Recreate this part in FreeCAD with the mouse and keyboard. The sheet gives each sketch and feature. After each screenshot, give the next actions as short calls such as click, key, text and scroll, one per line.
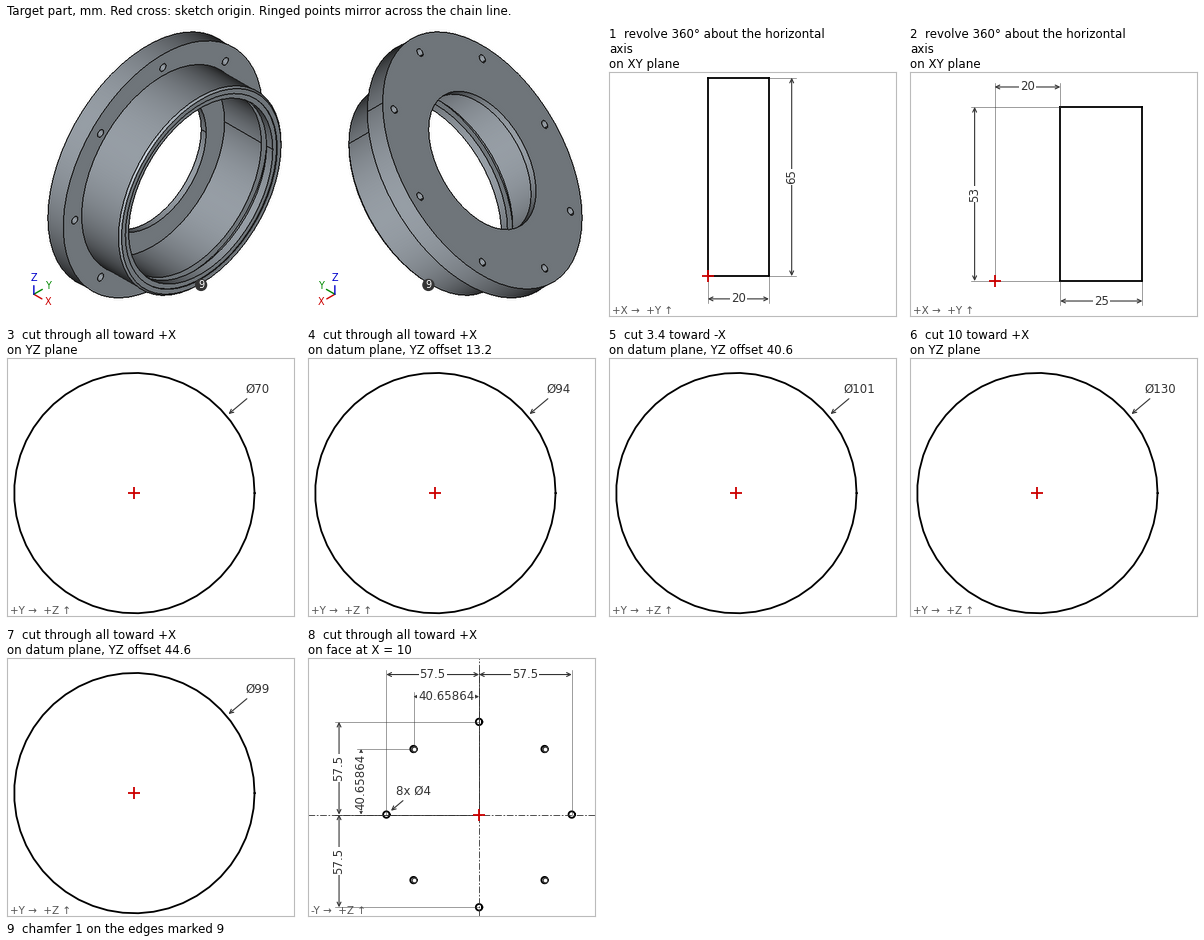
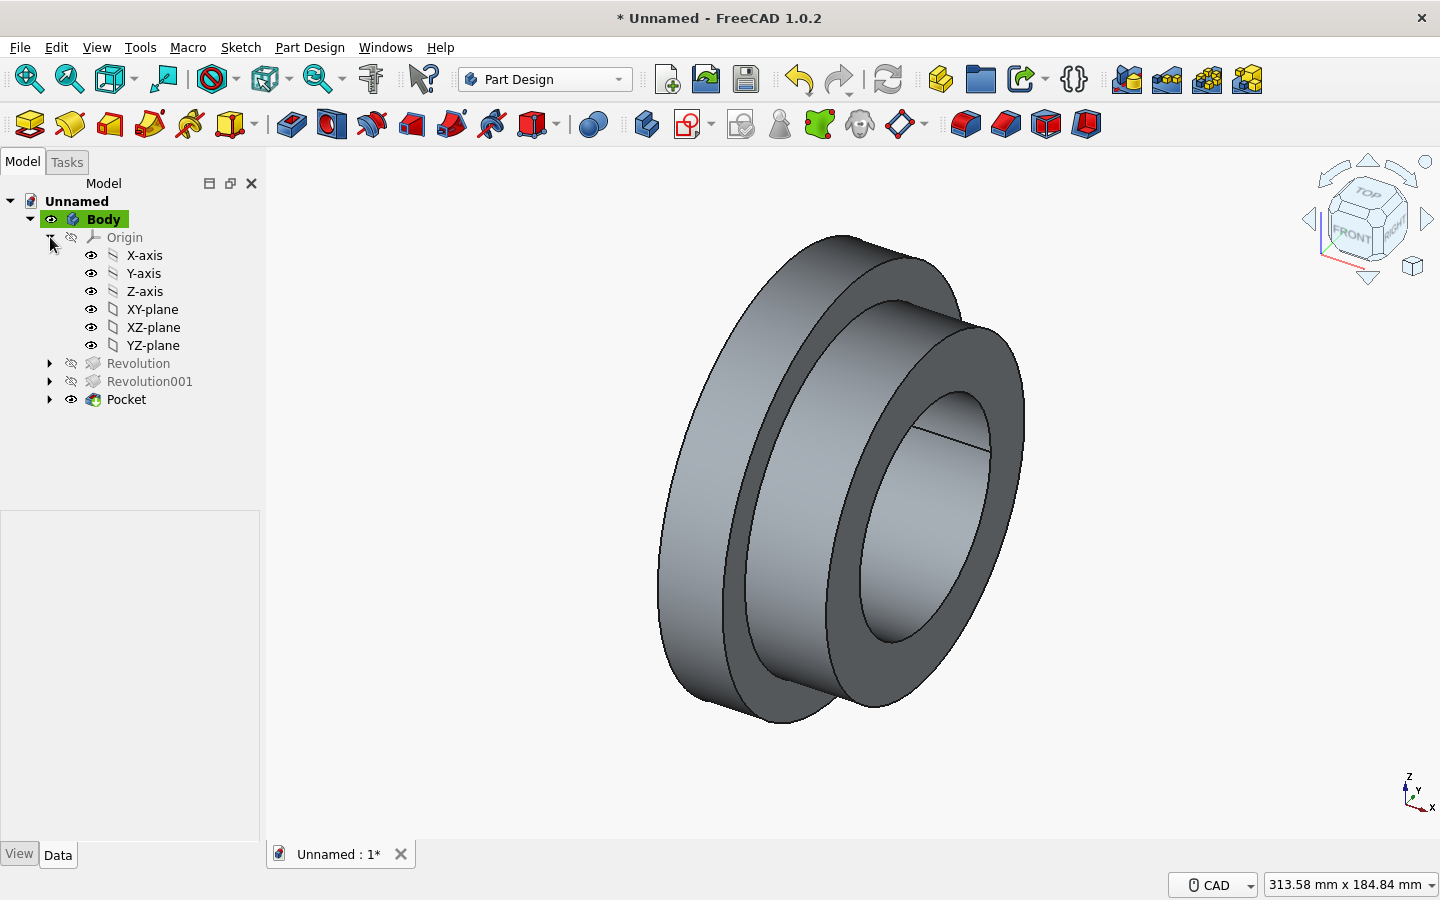
click(136, 345)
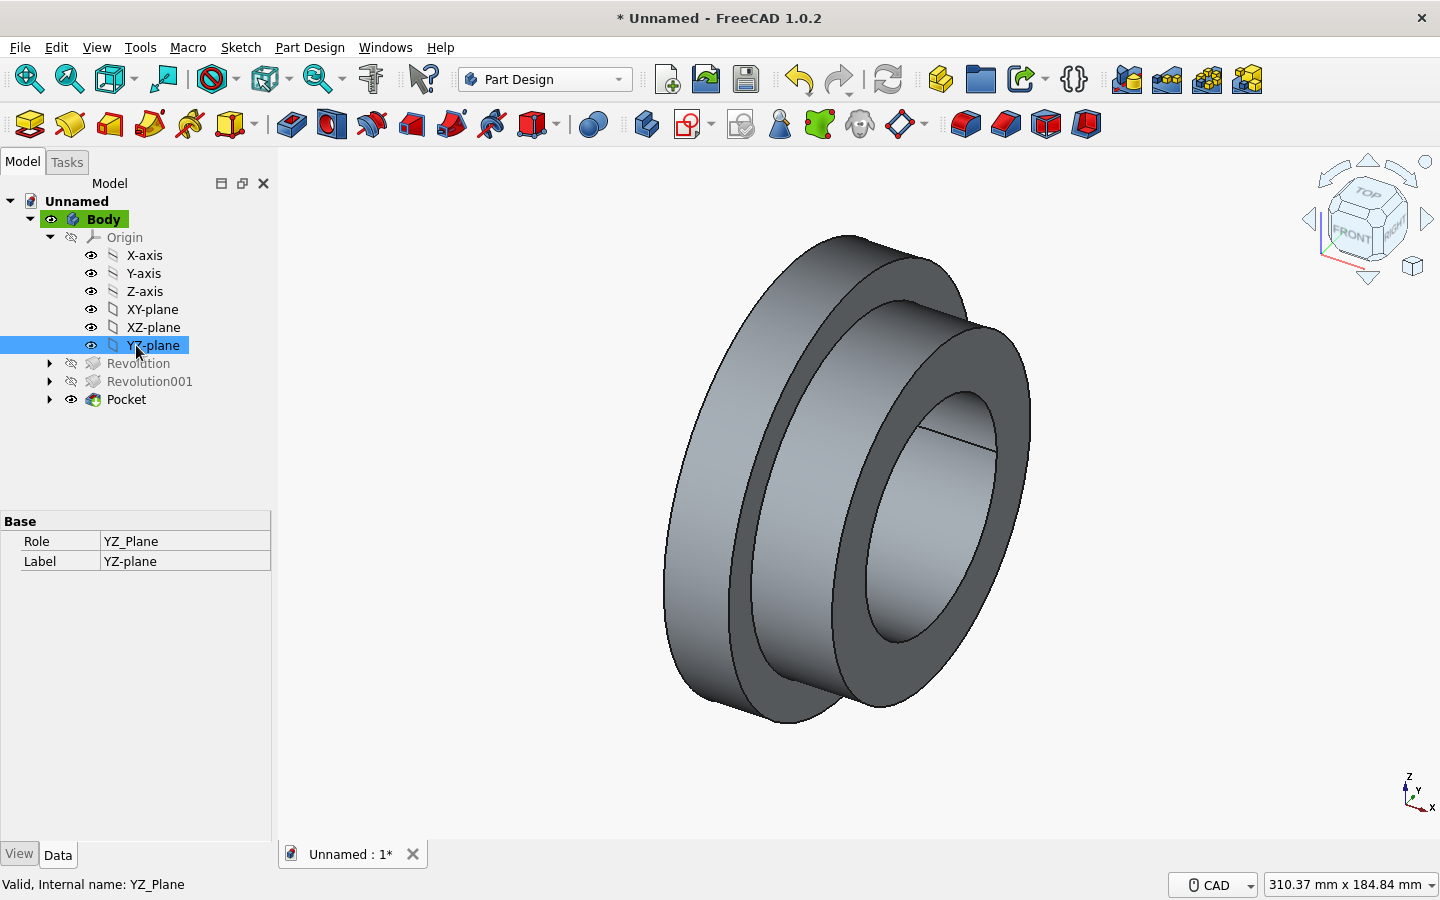
click(900, 124)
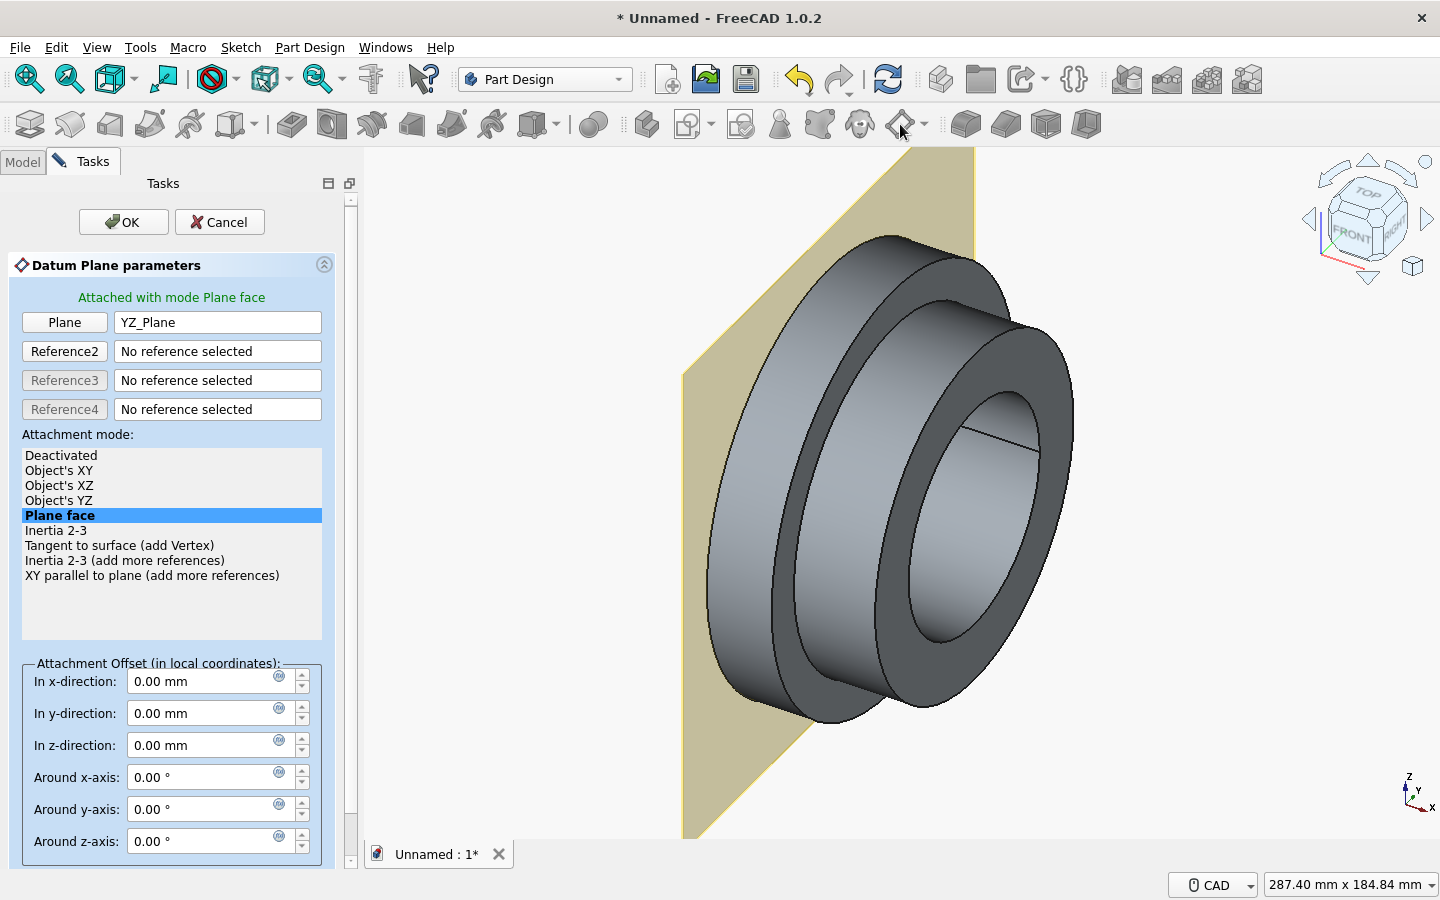
triple_click(210, 745)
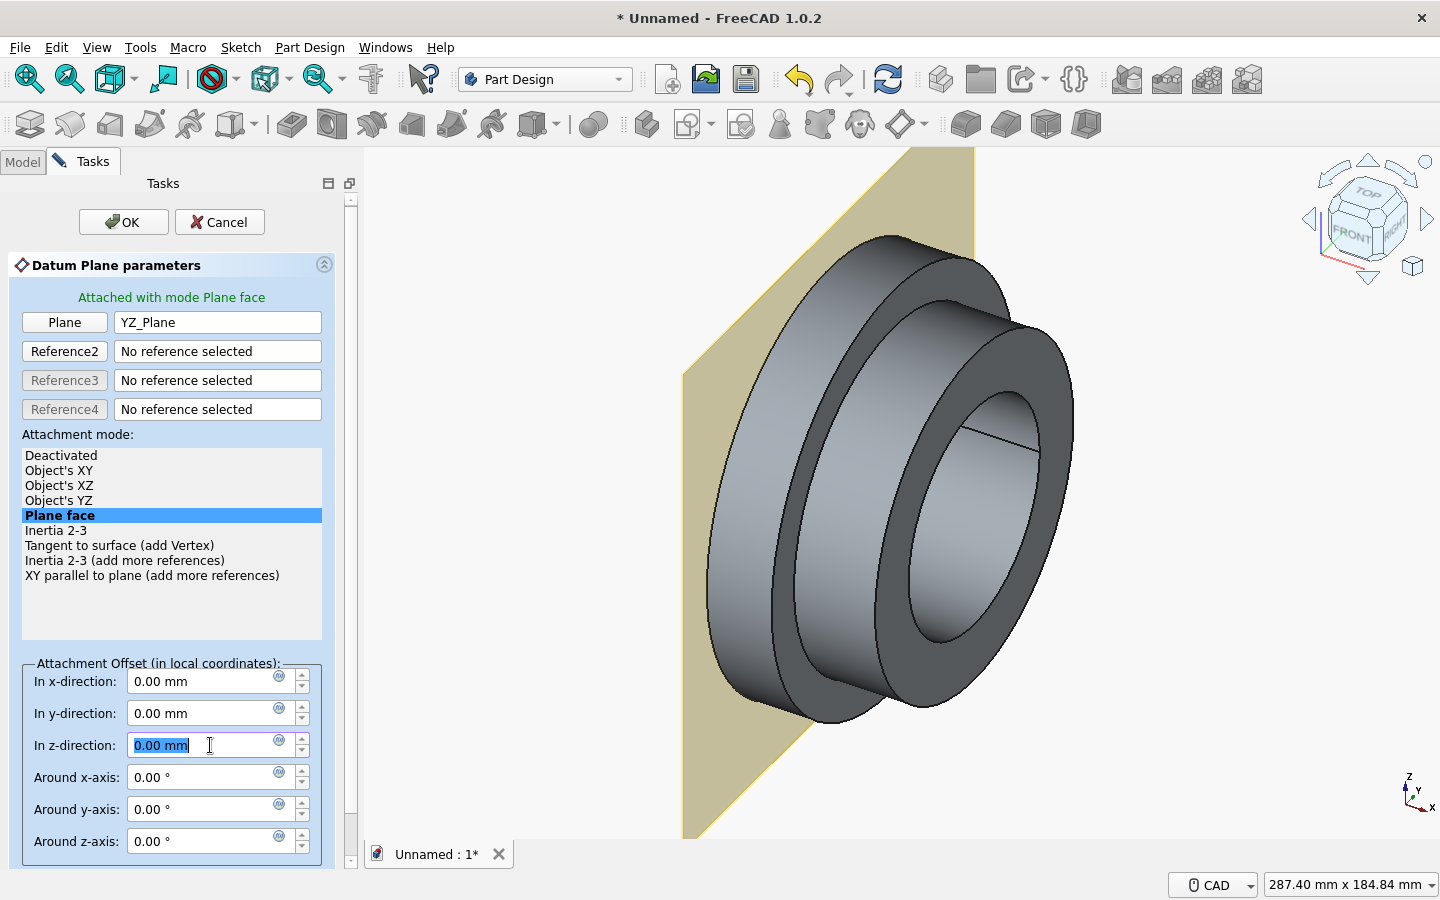
text(13.2)
key(Tab)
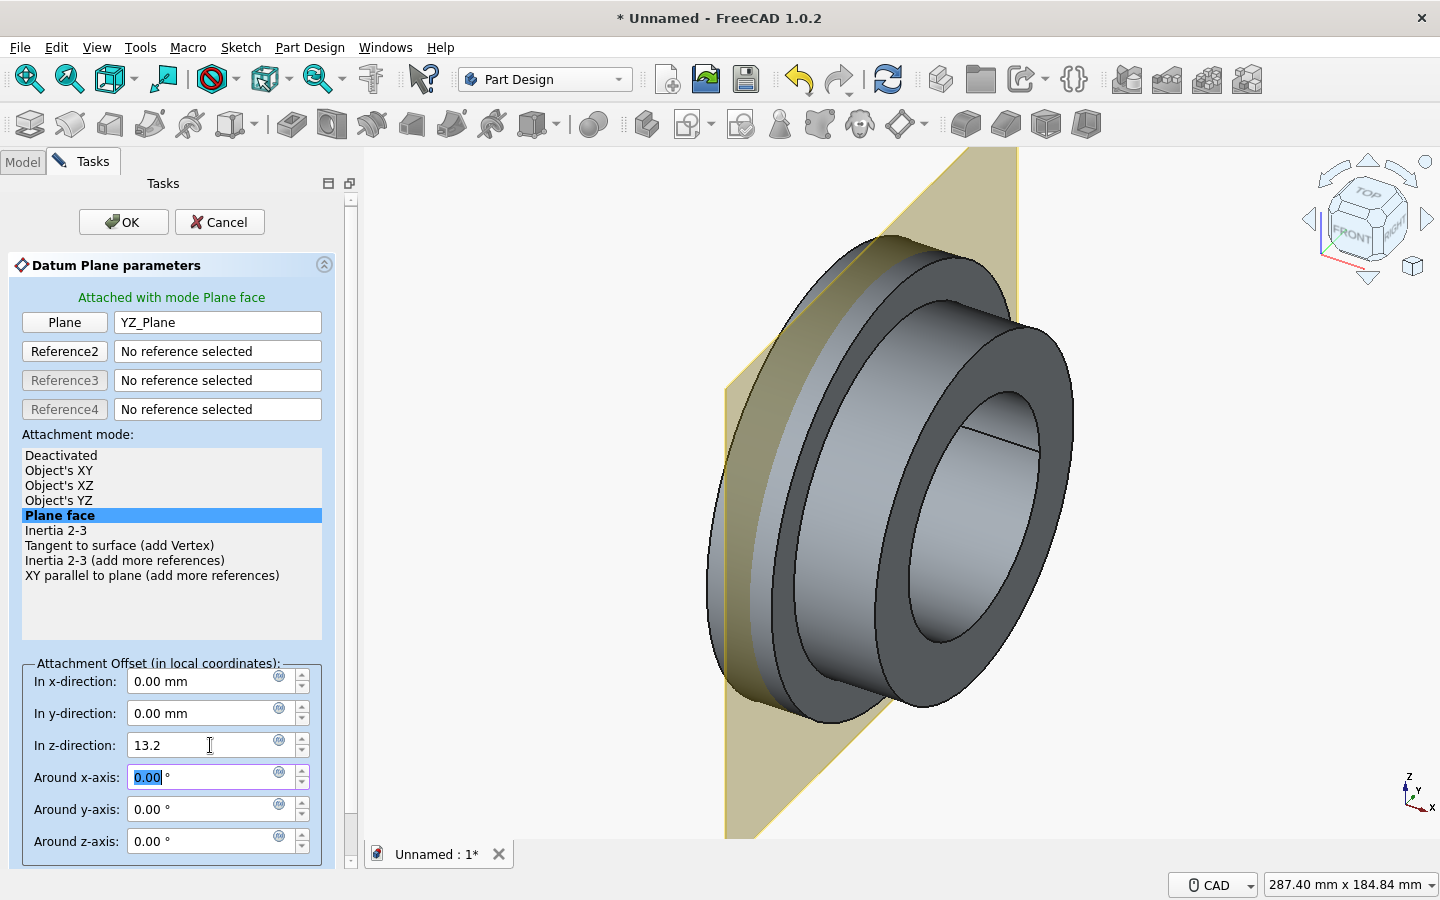
click(124, 222)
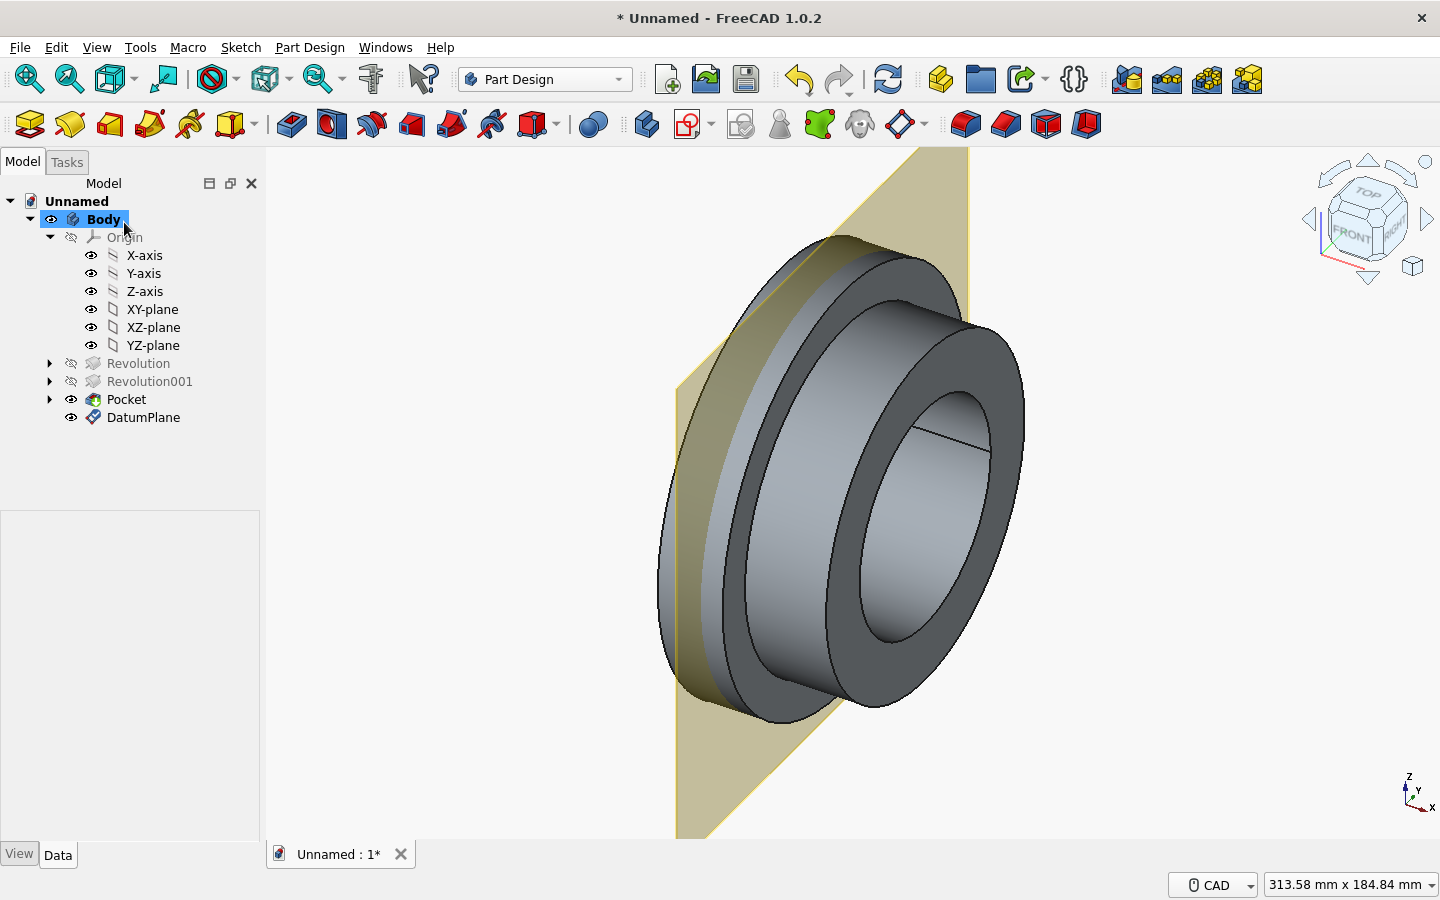
click(116, 417)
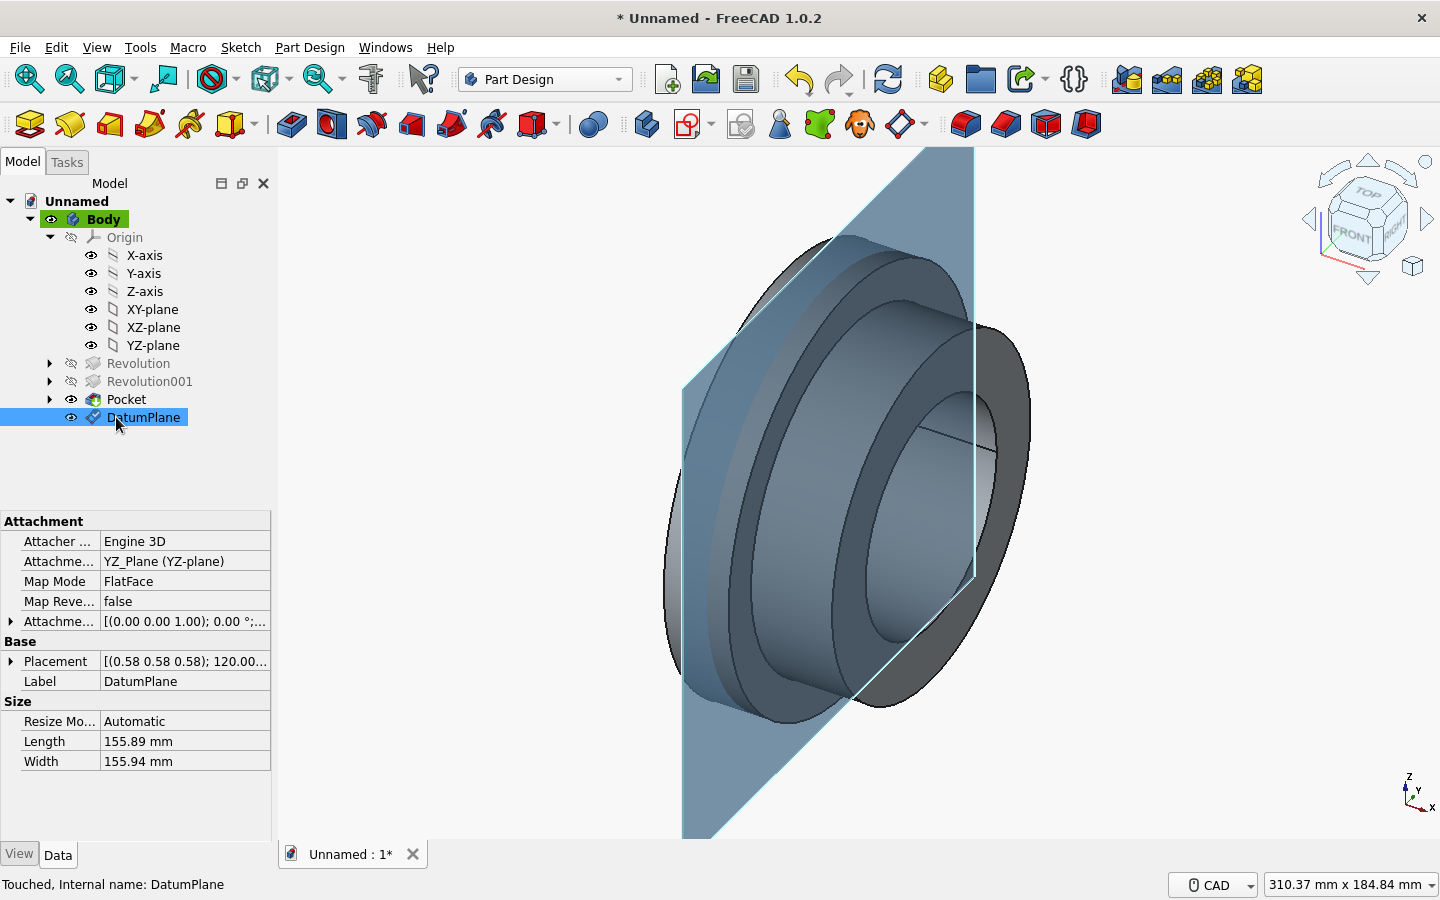
click(688, 124)